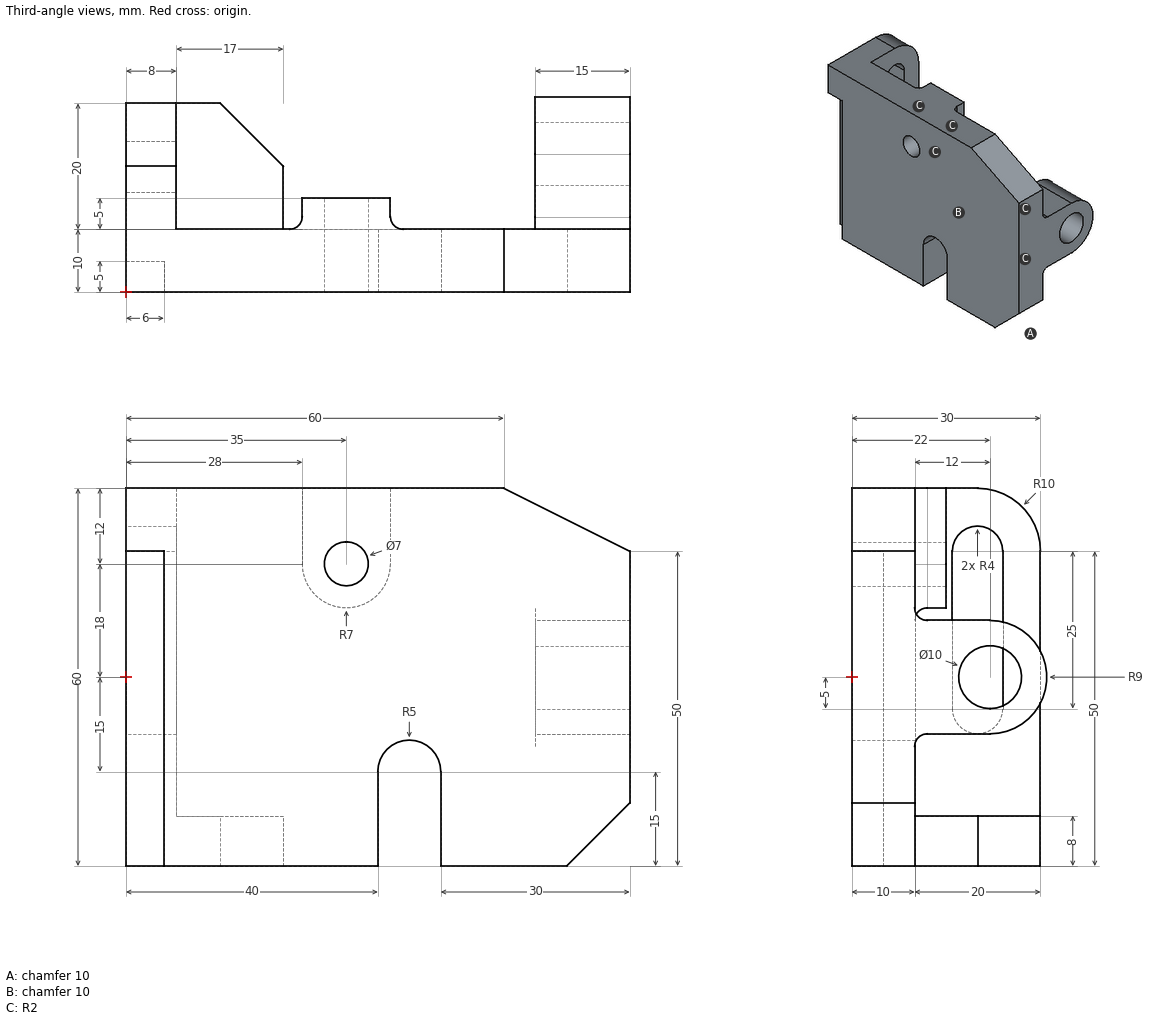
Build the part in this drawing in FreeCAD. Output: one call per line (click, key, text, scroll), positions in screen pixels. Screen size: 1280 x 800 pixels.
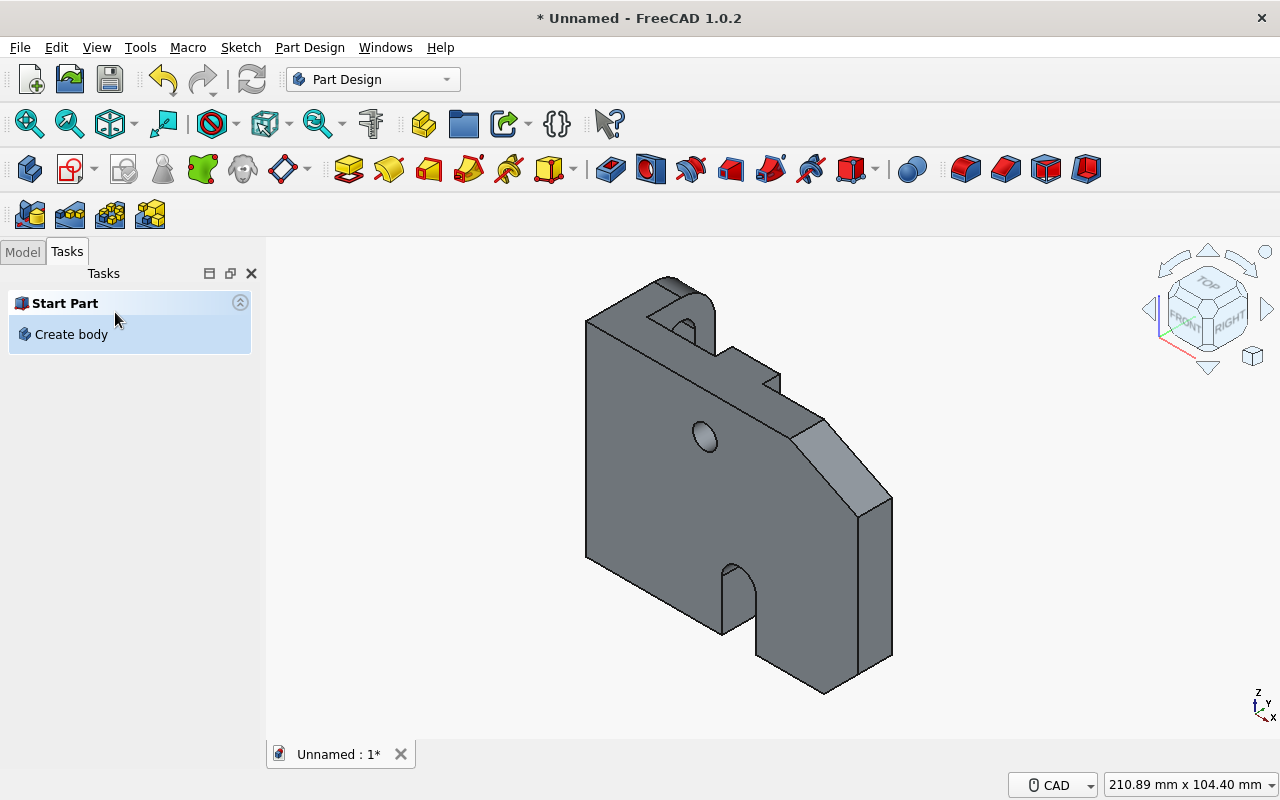
click(875, 608)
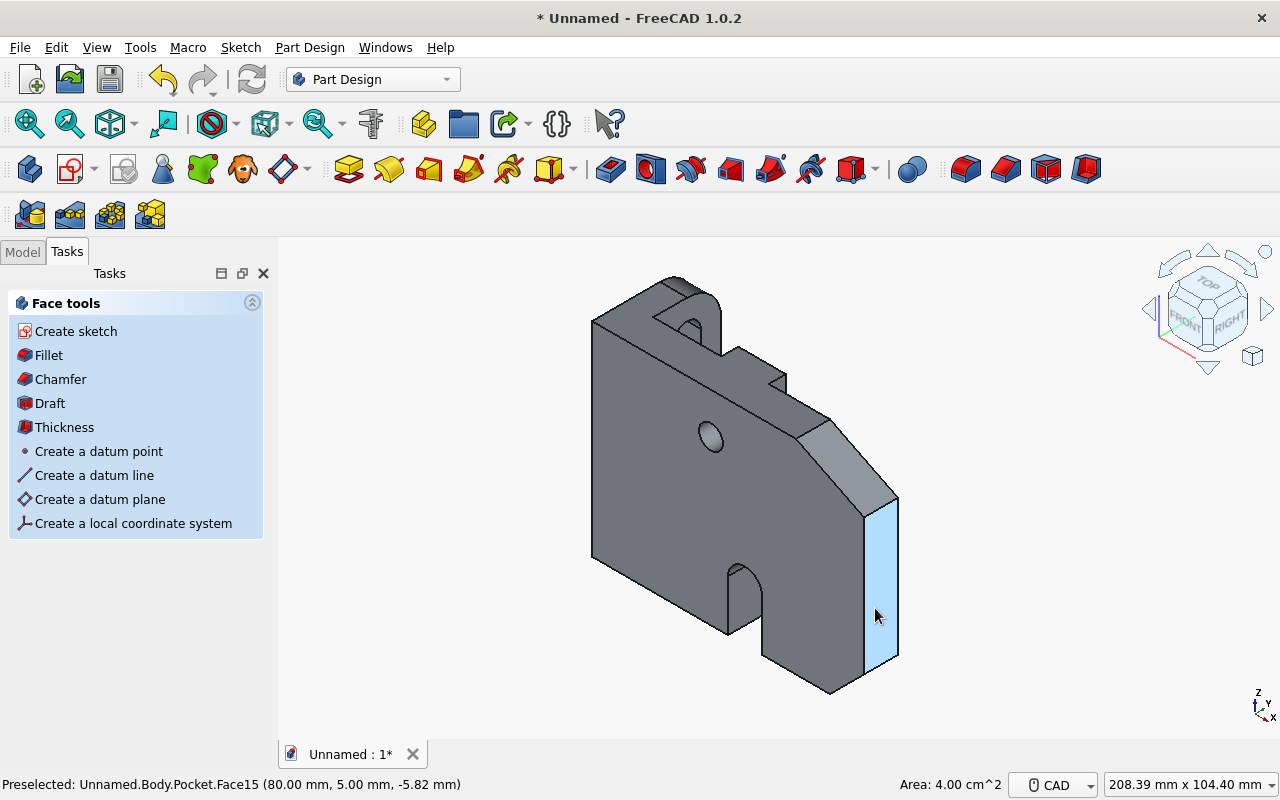
click(70, 170)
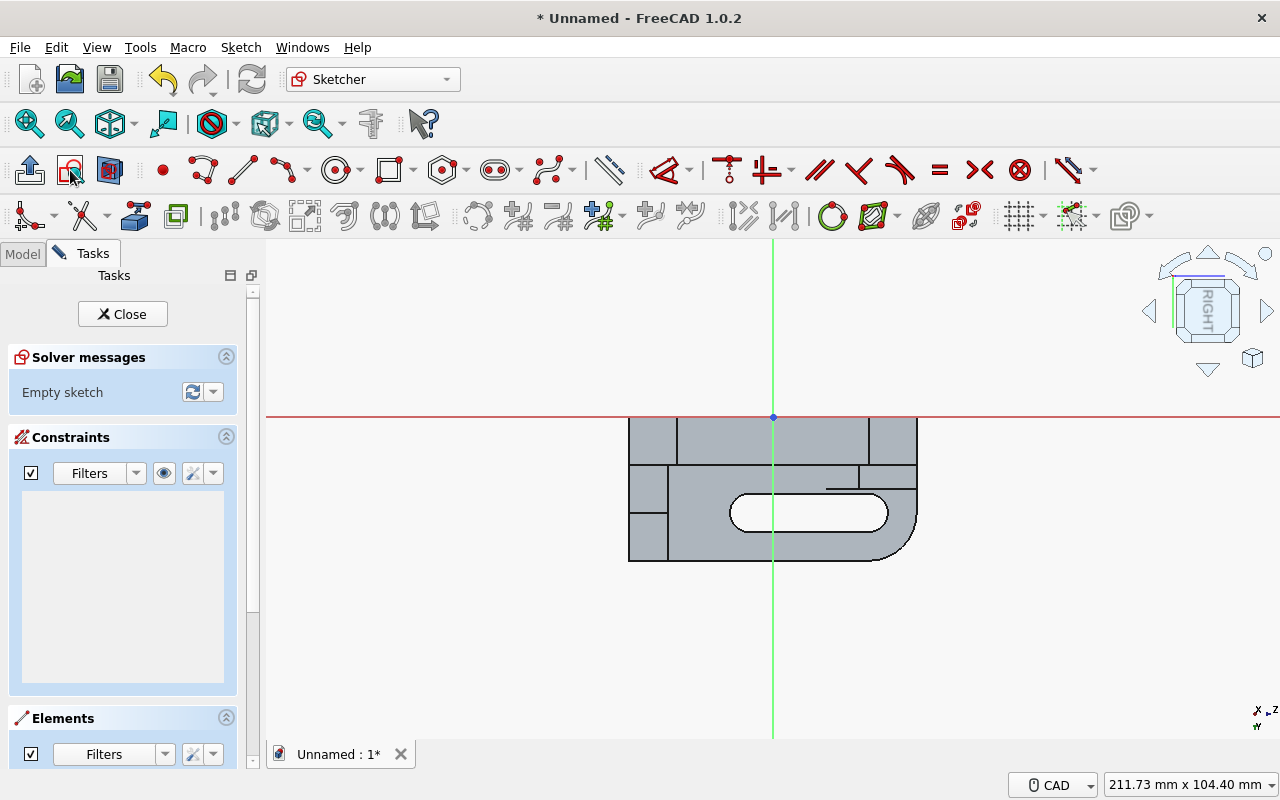
scroll(829, 493, up, 4)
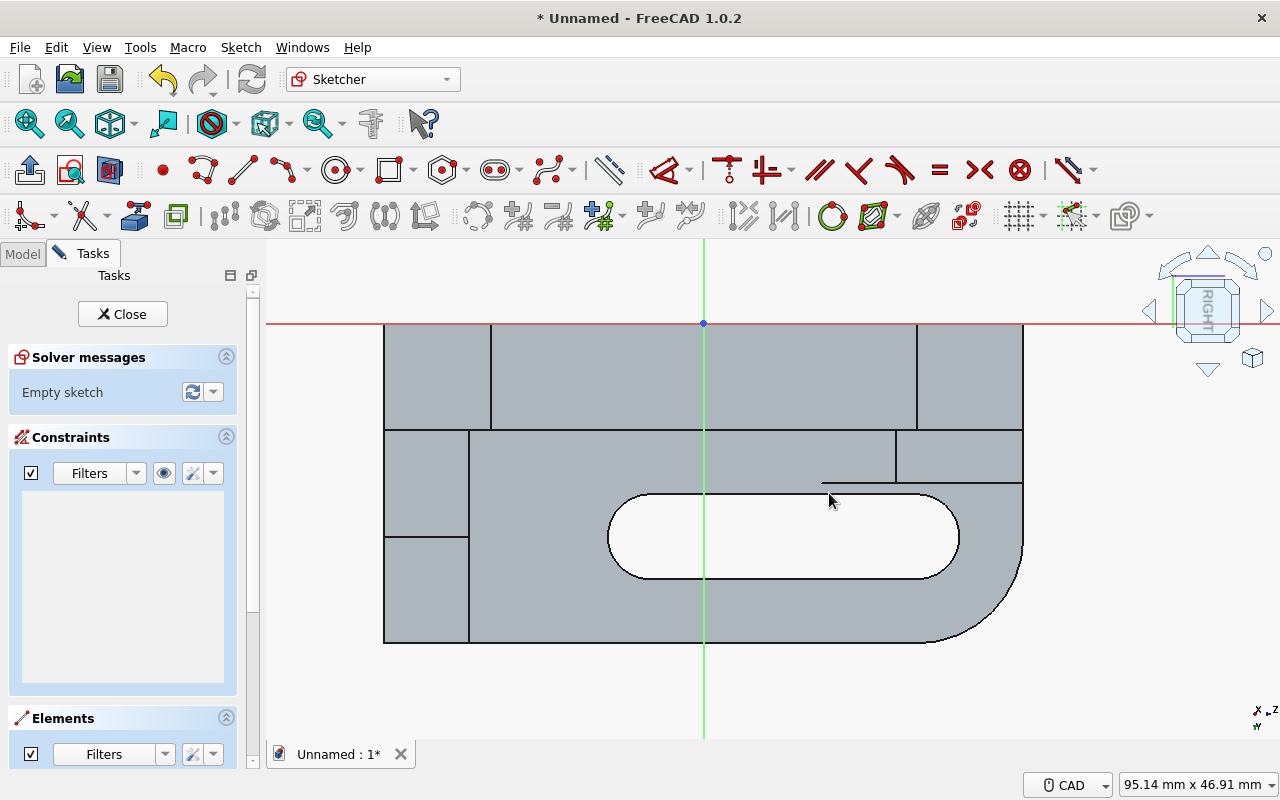
click(204, 170)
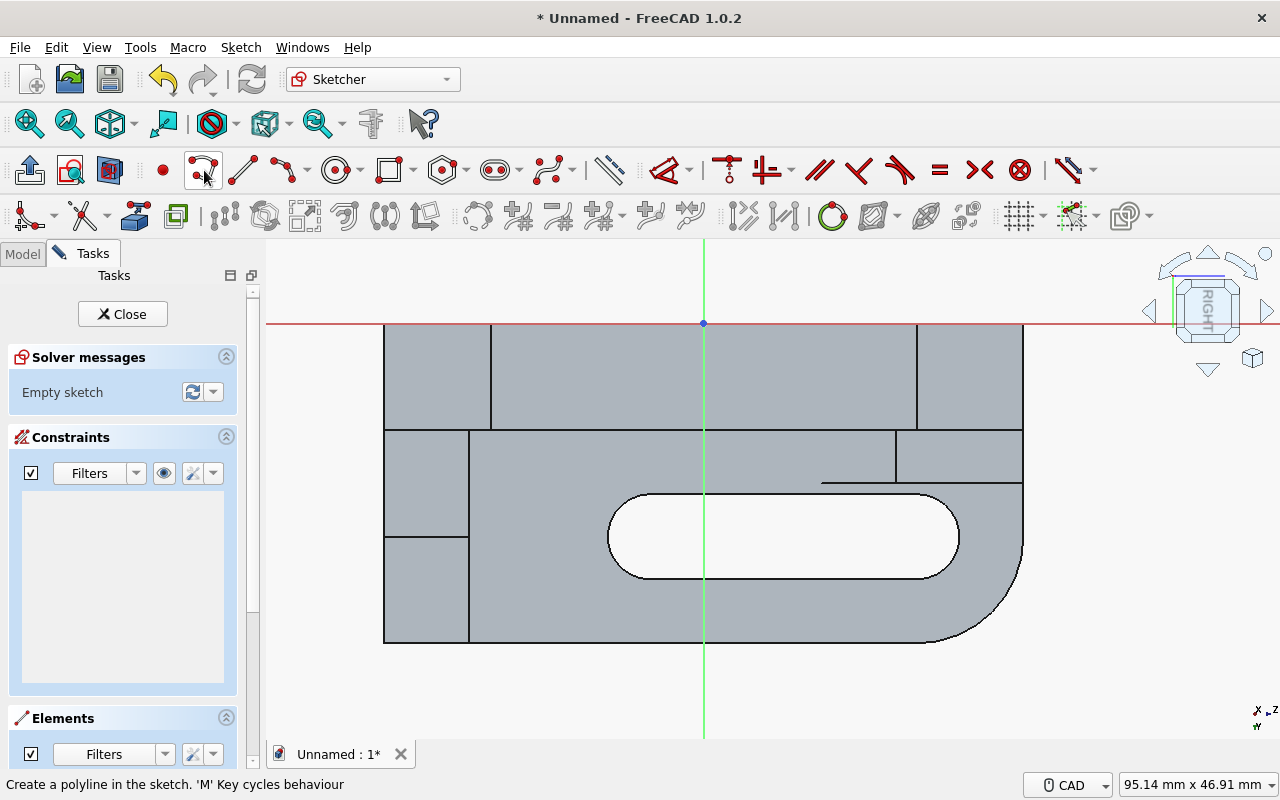
click(800, 558)
click(800, 430)
click(608, 430)
click(608, 558)
right_click(608, 558)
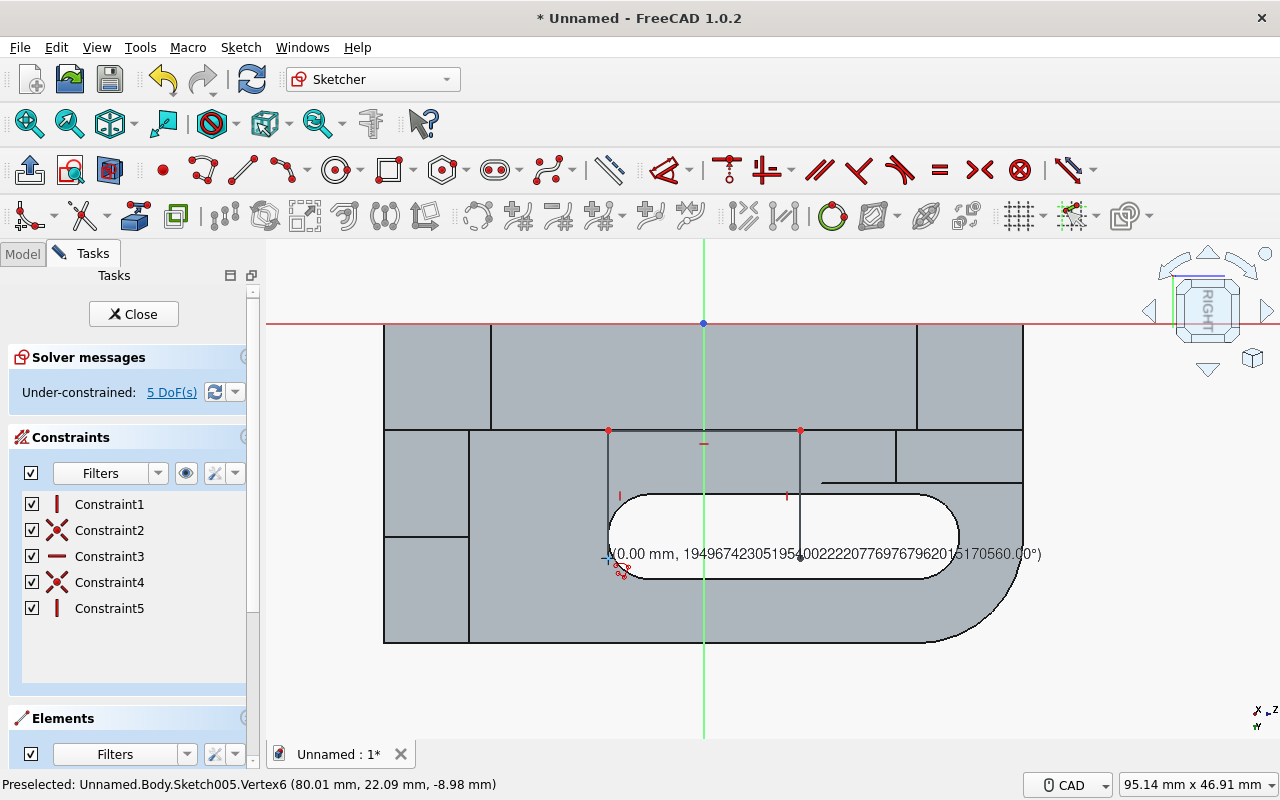
click(284, 170)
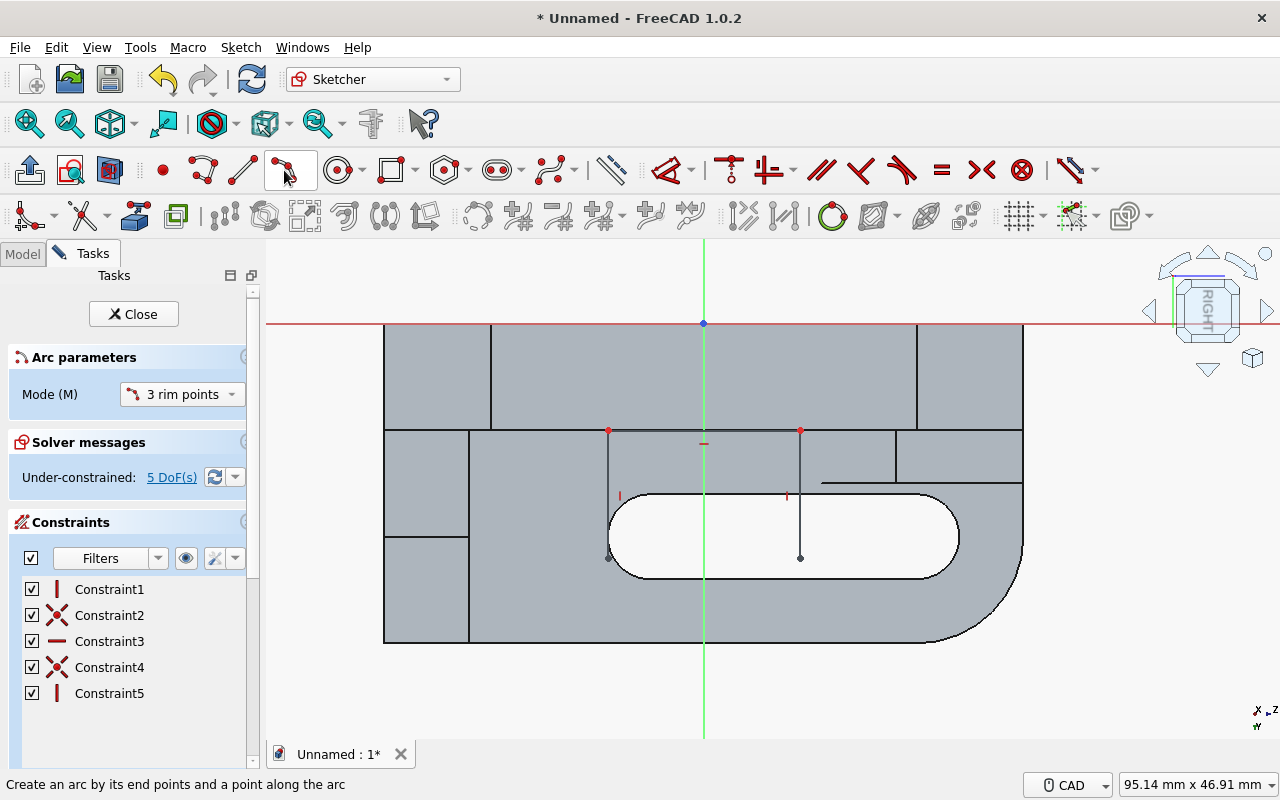
click(608, 559)
click(800, 559)
click(674, 649)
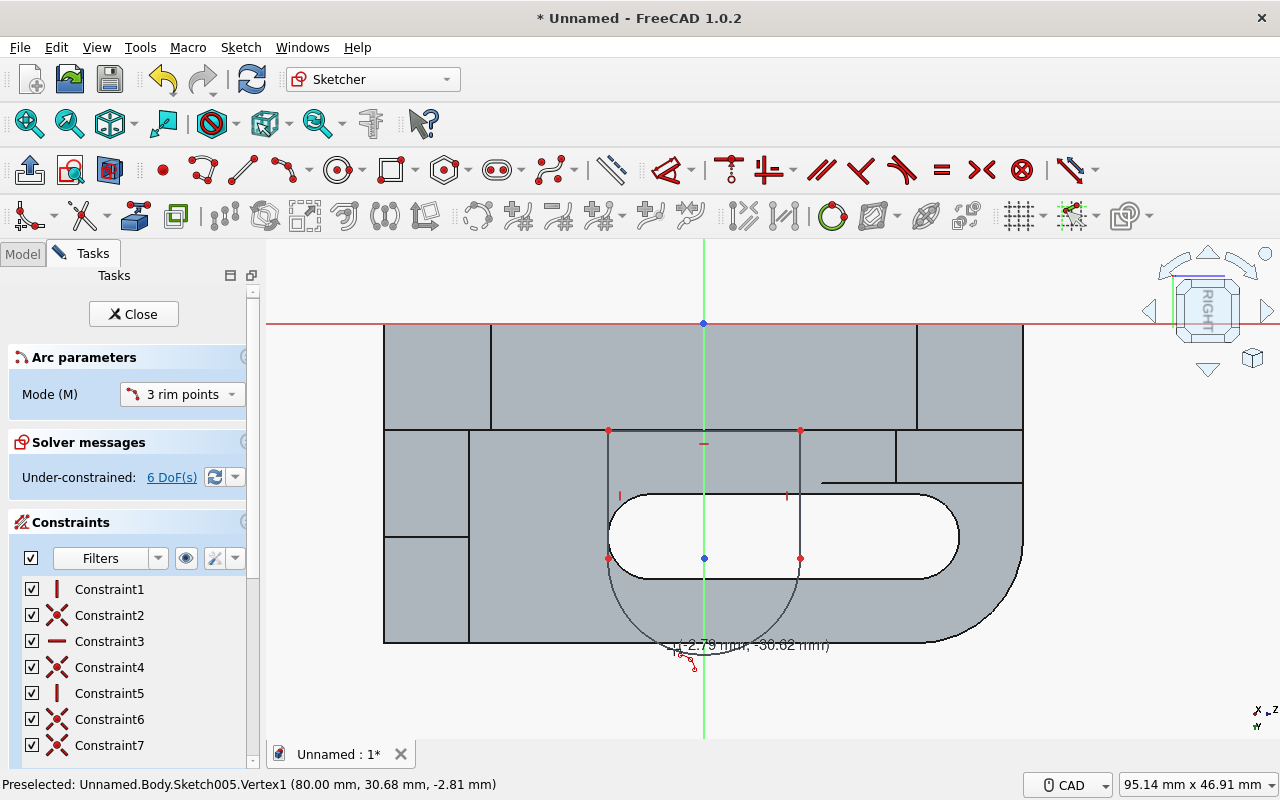
click(338, 170)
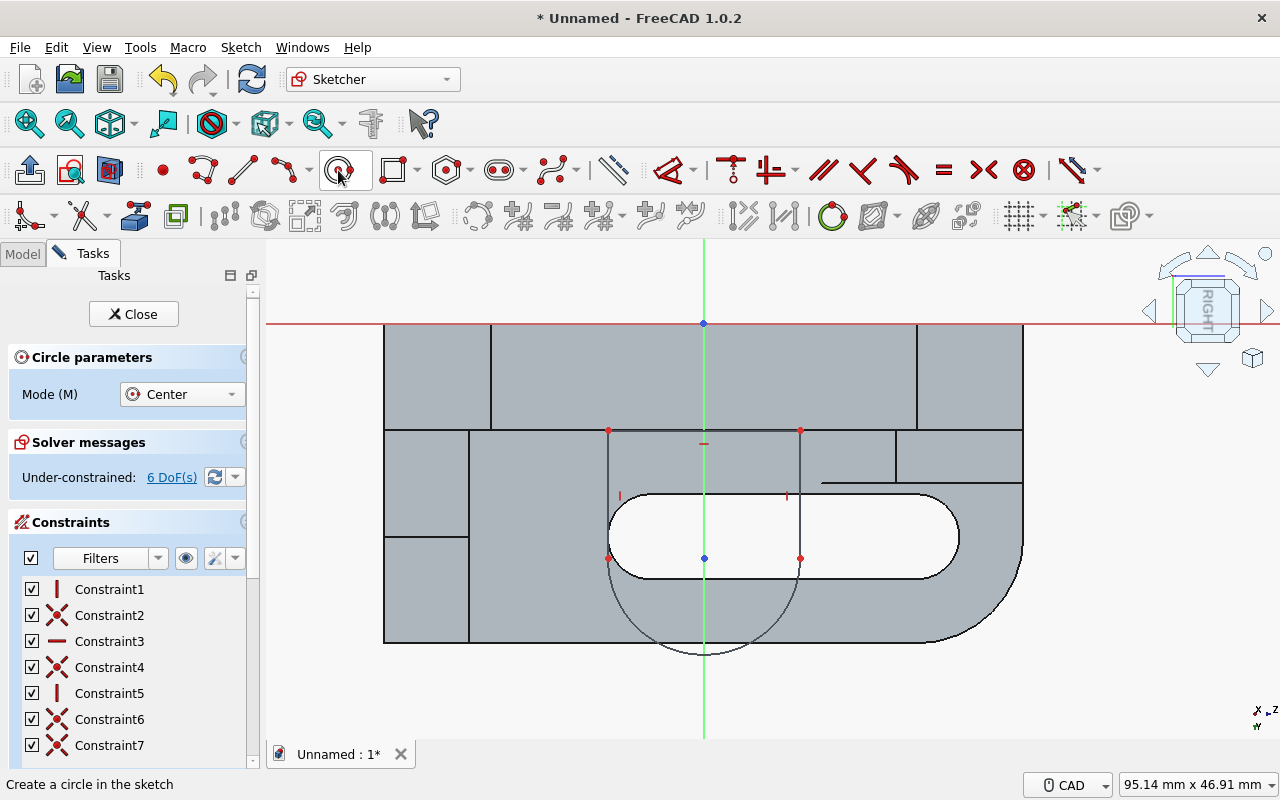
click(704, 558)
click(741, 520)
key(Escape)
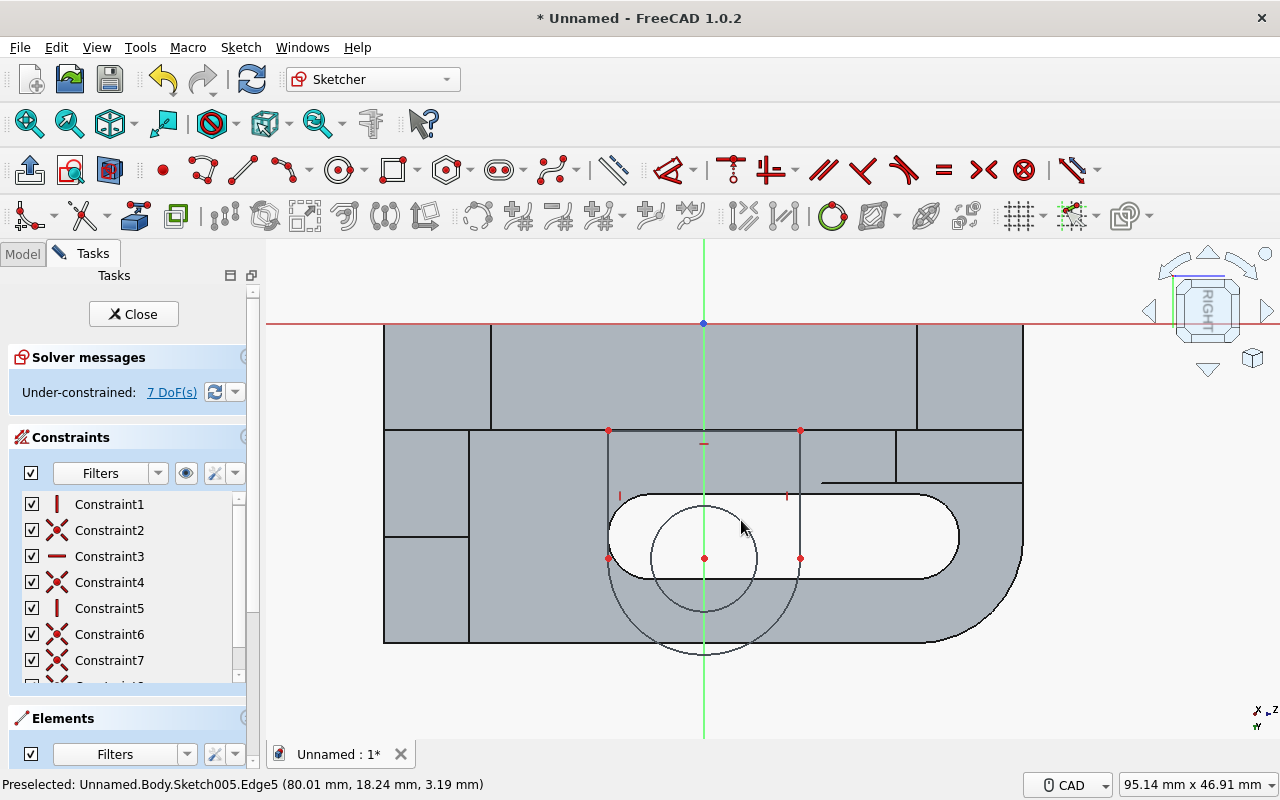
click(800, 521)